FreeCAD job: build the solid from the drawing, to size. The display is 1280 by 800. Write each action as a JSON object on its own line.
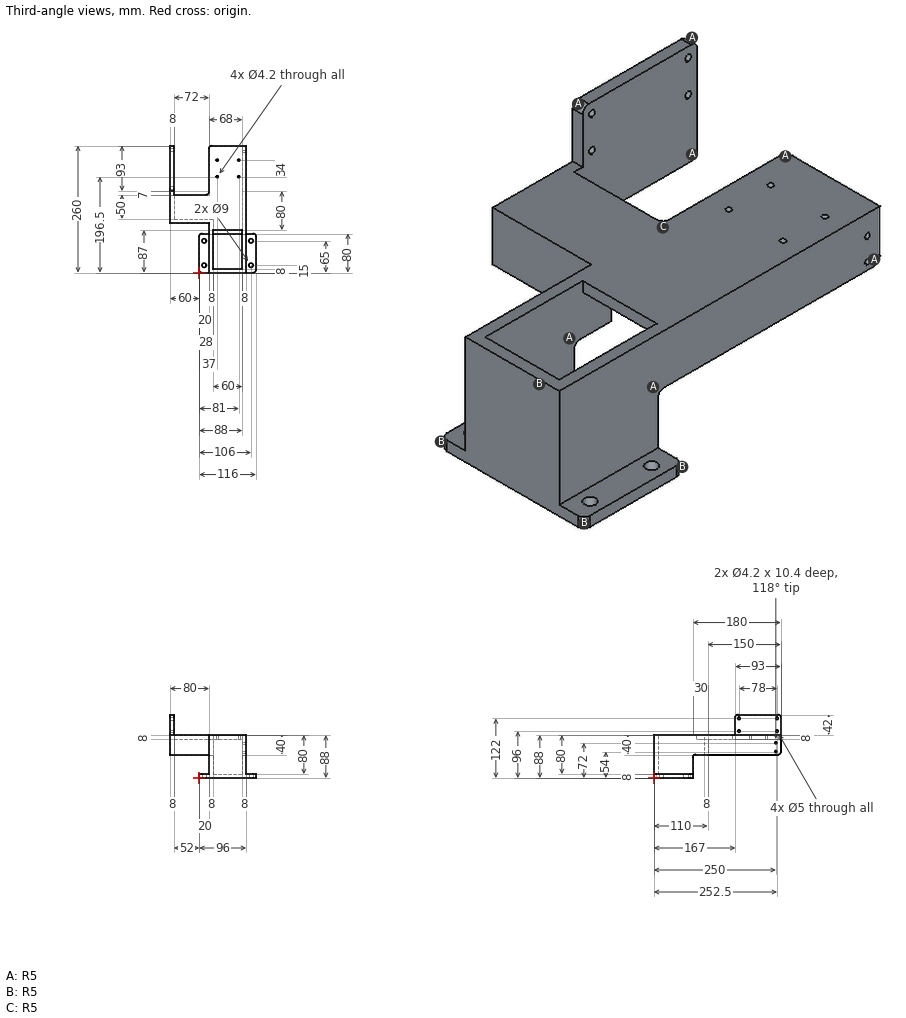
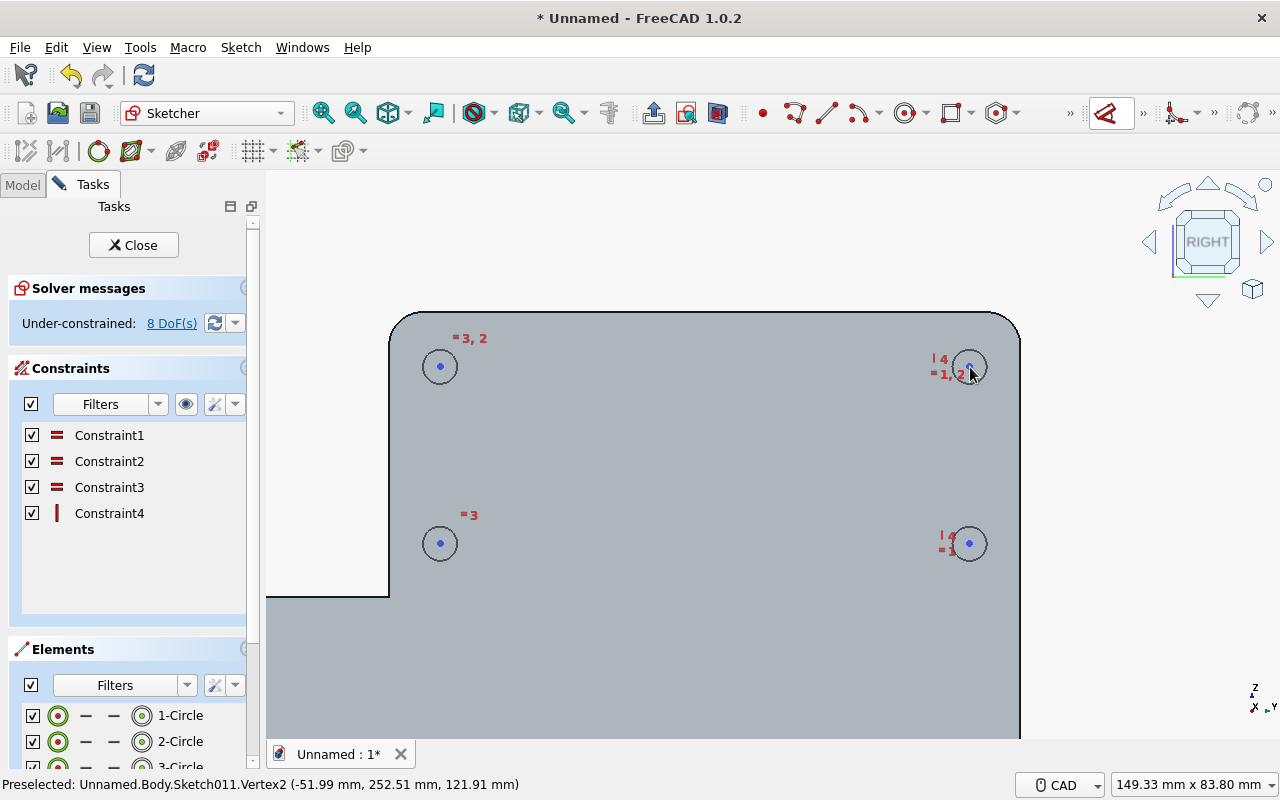
{"action": "left_click", "coordinate": [970, 367]}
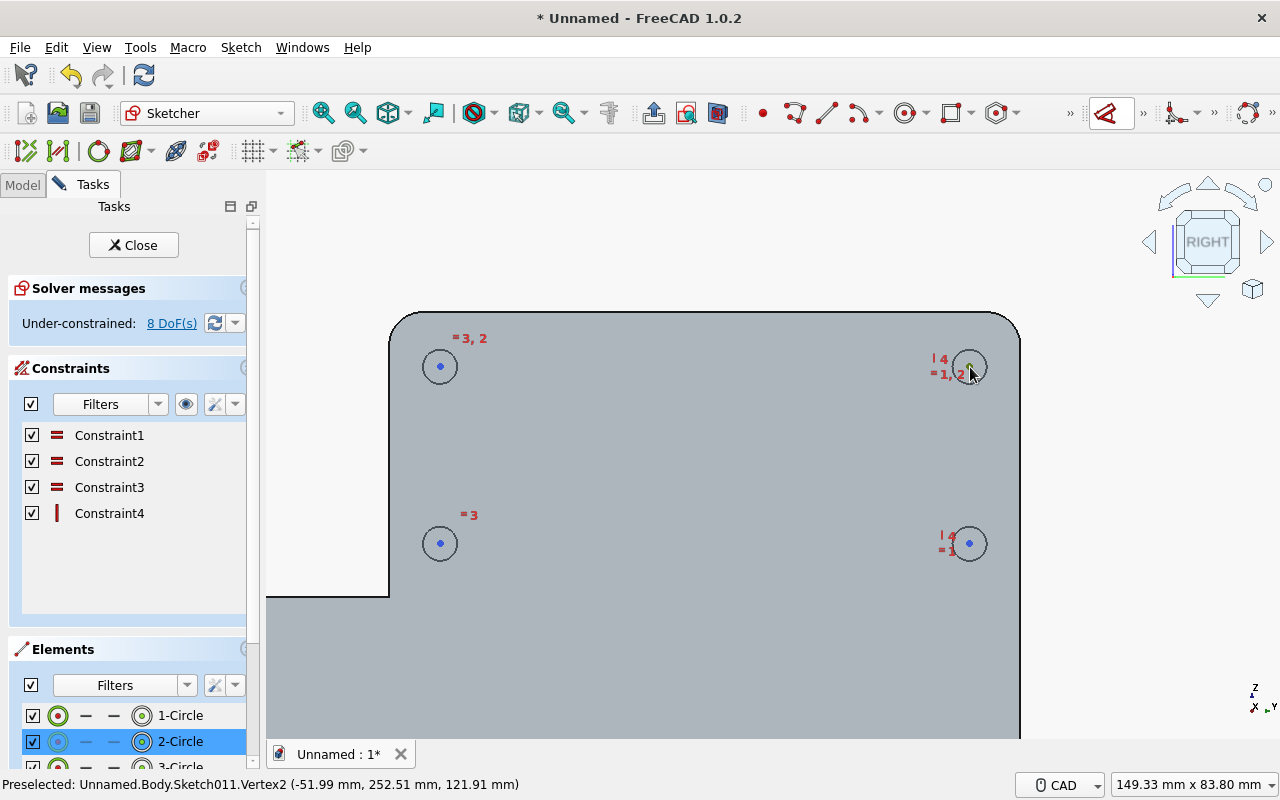
{"action": "left_click", "coordinate": [440, 367]}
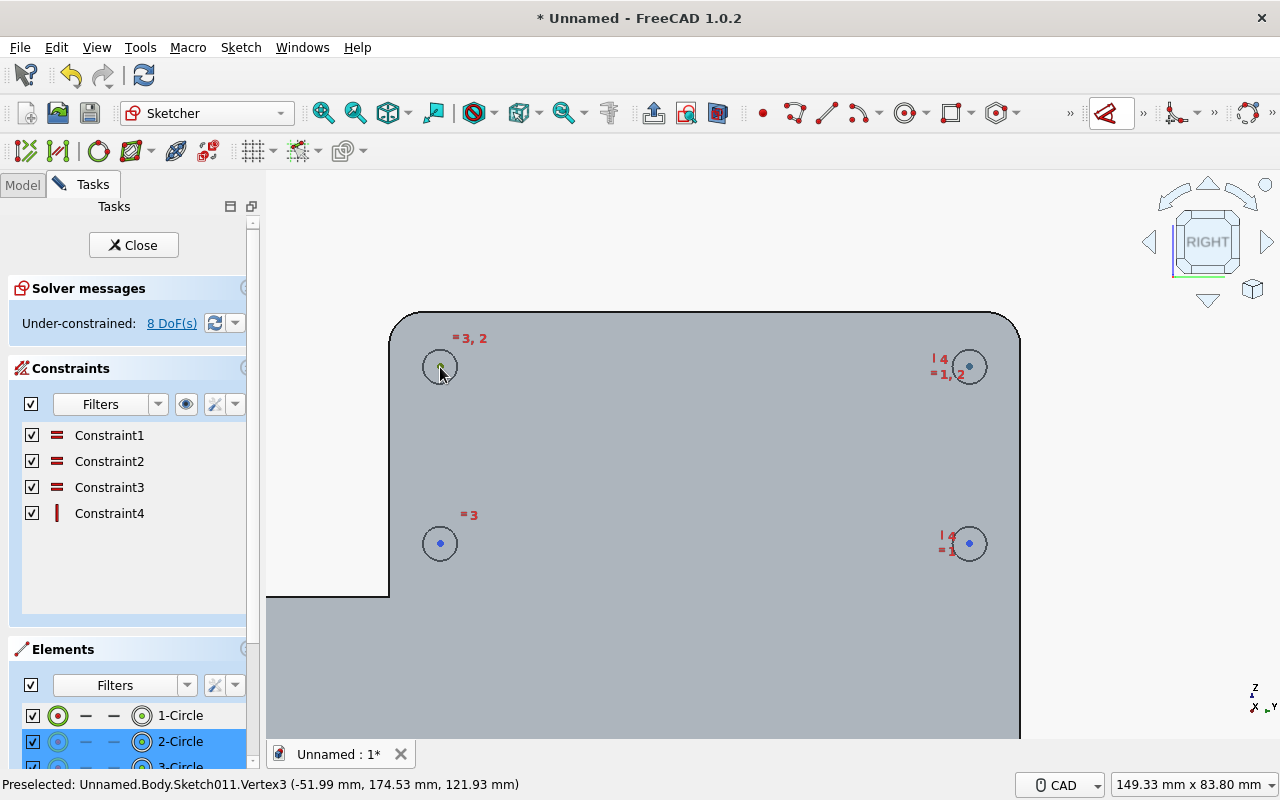
{"action": "key", "text": "h"}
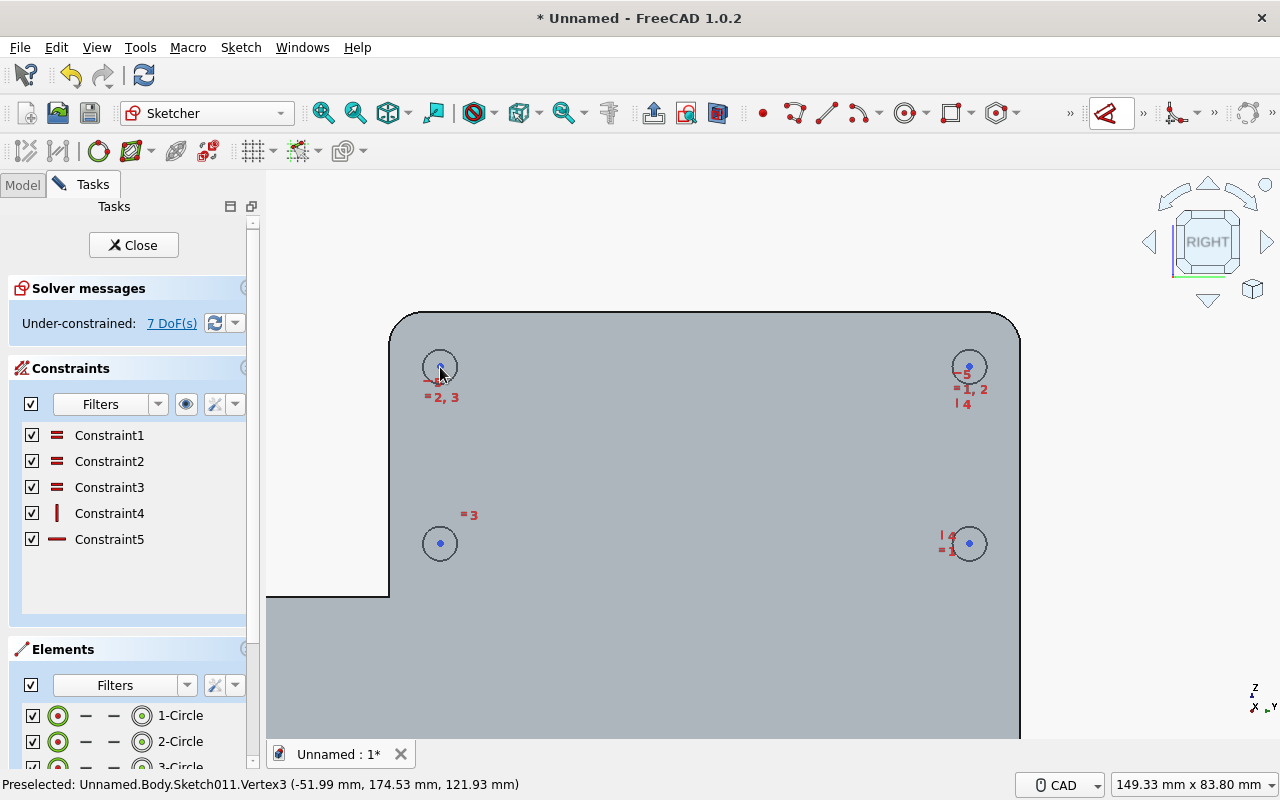
{"action": "left_click", "coordinate": [440, 367]}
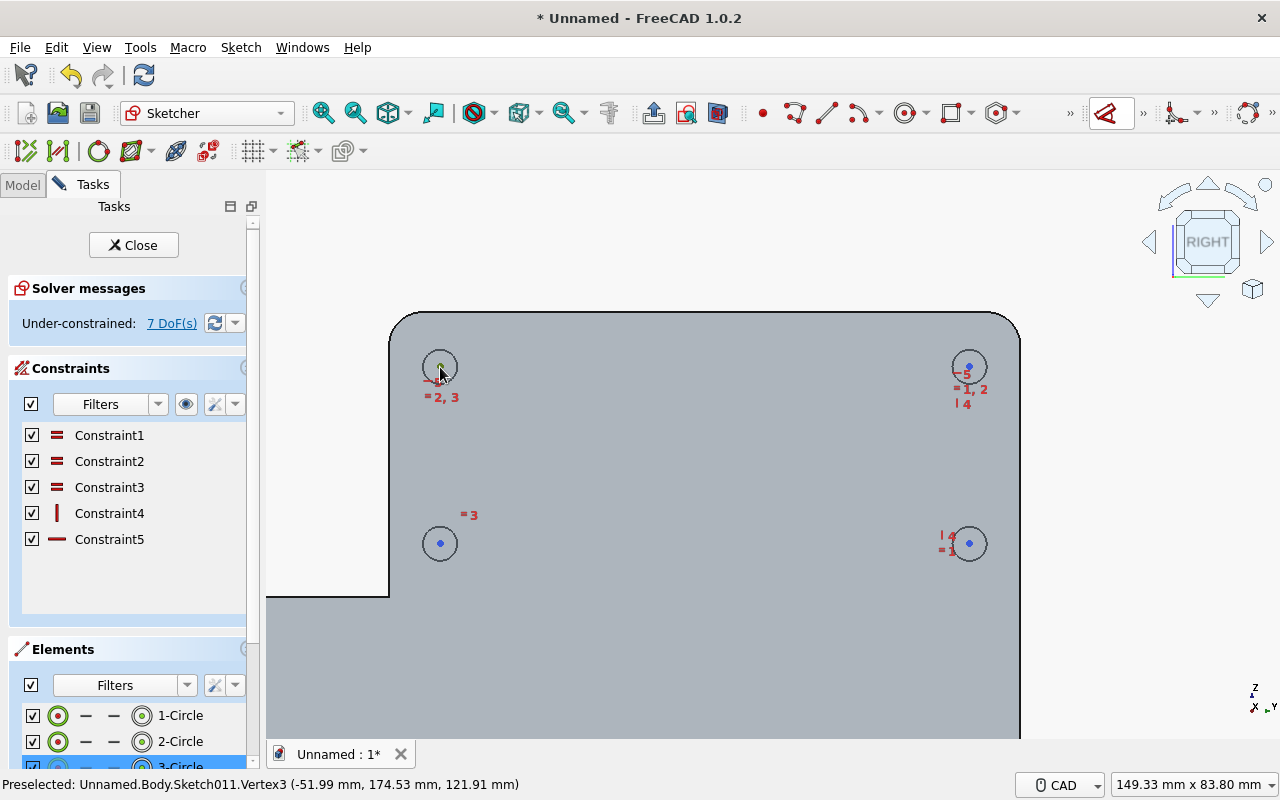
{"action": "left_click", "coordinate": [440, 544]}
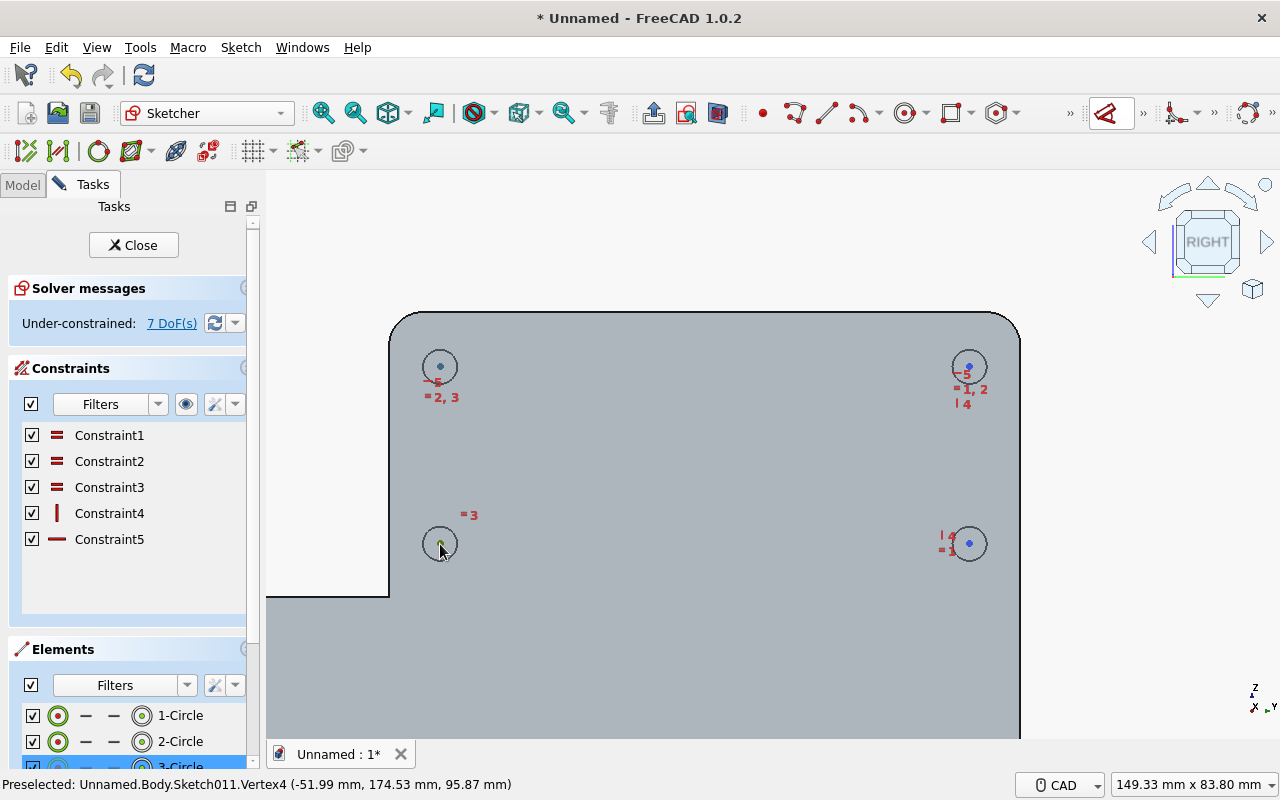
{"action": "key", "text": "v"}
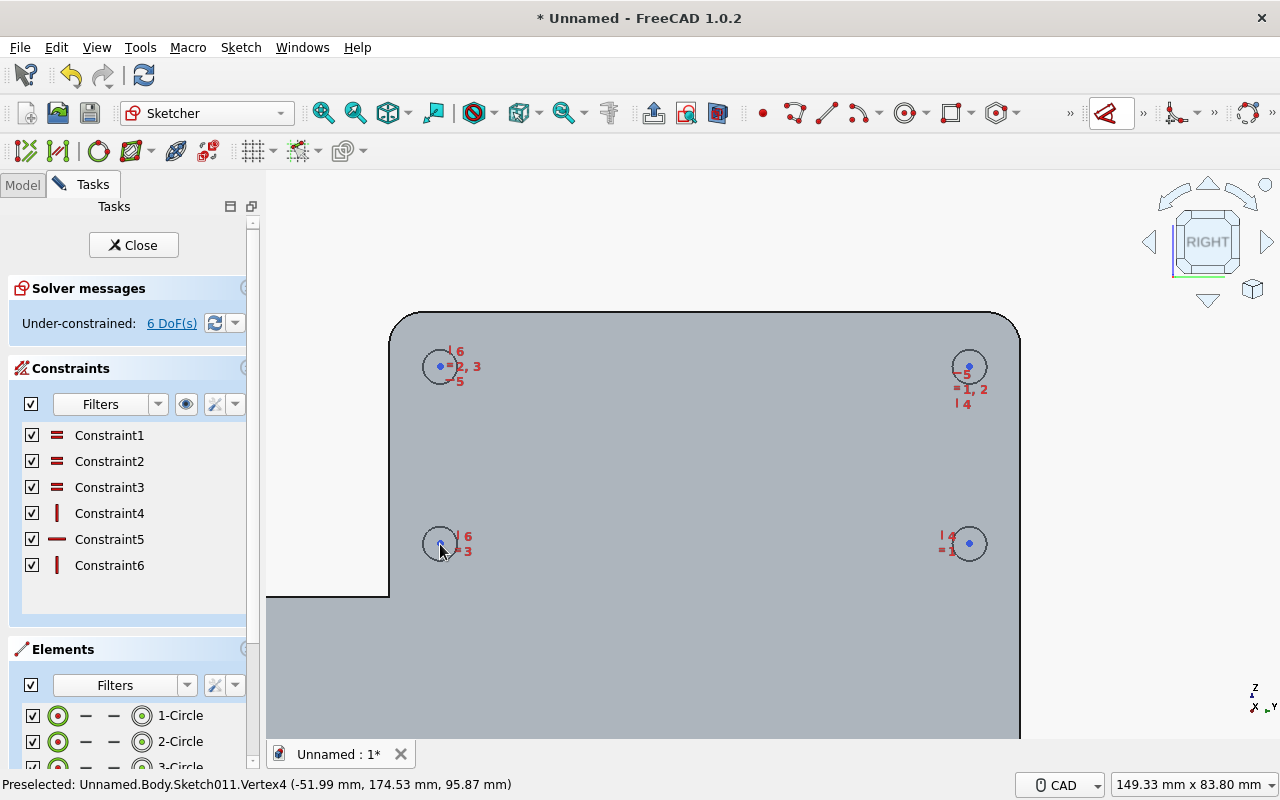
{"action": "left_click", "coordinate": [970, 544]}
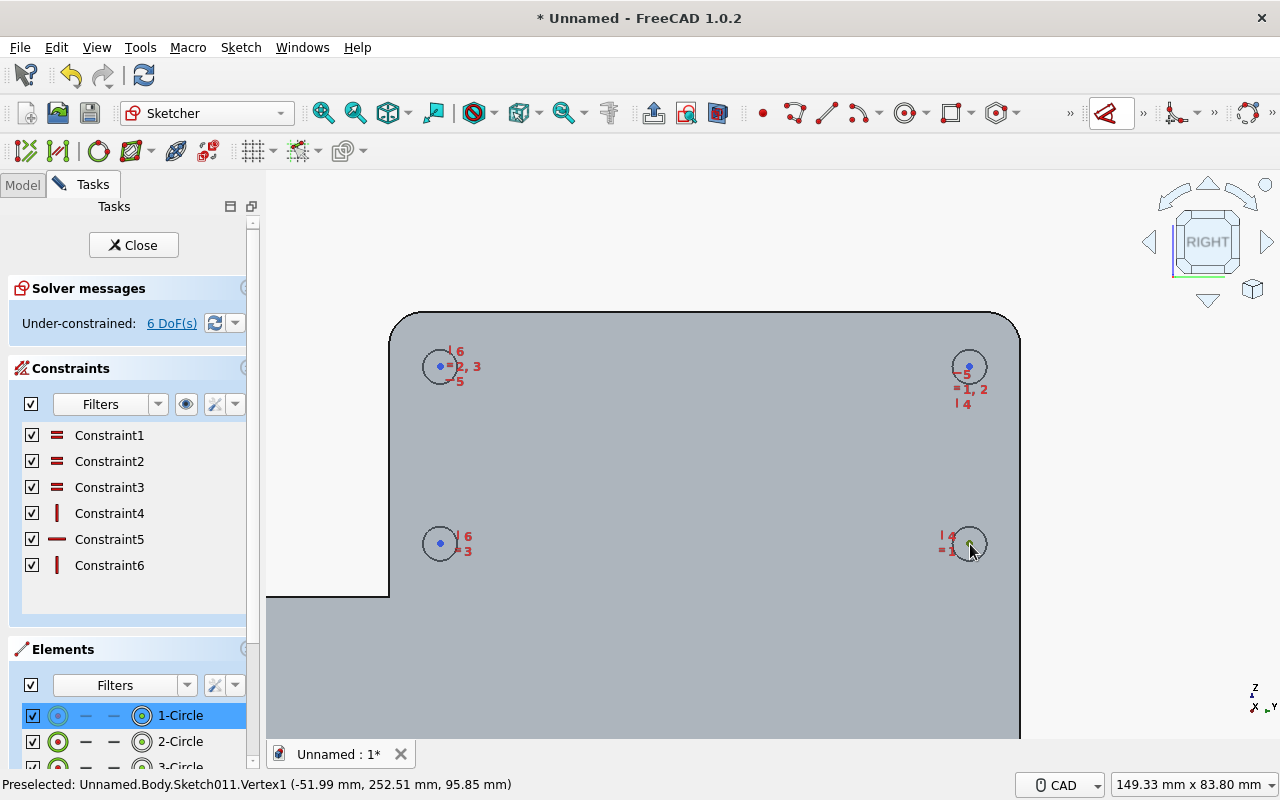
{"action": "left_click", "coordinate": [440, 544]}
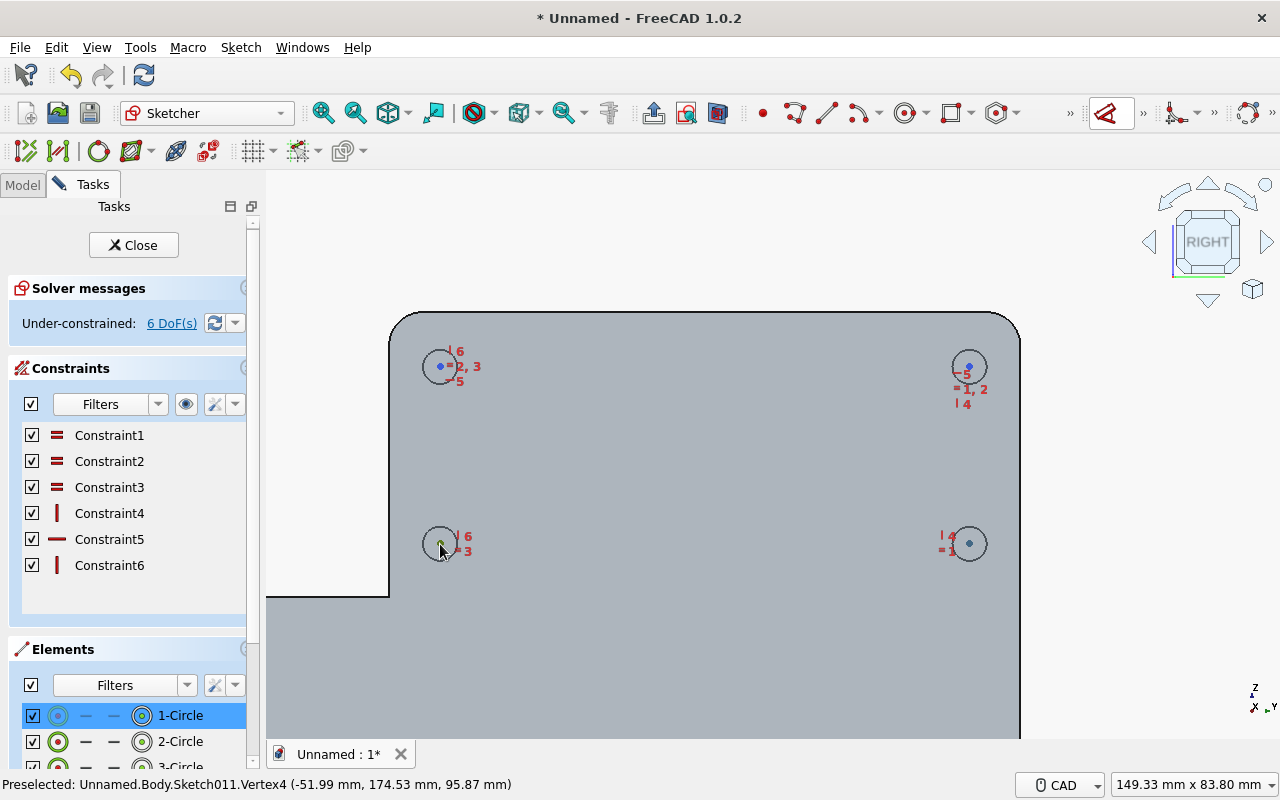
{"action": "key", "text": "h"}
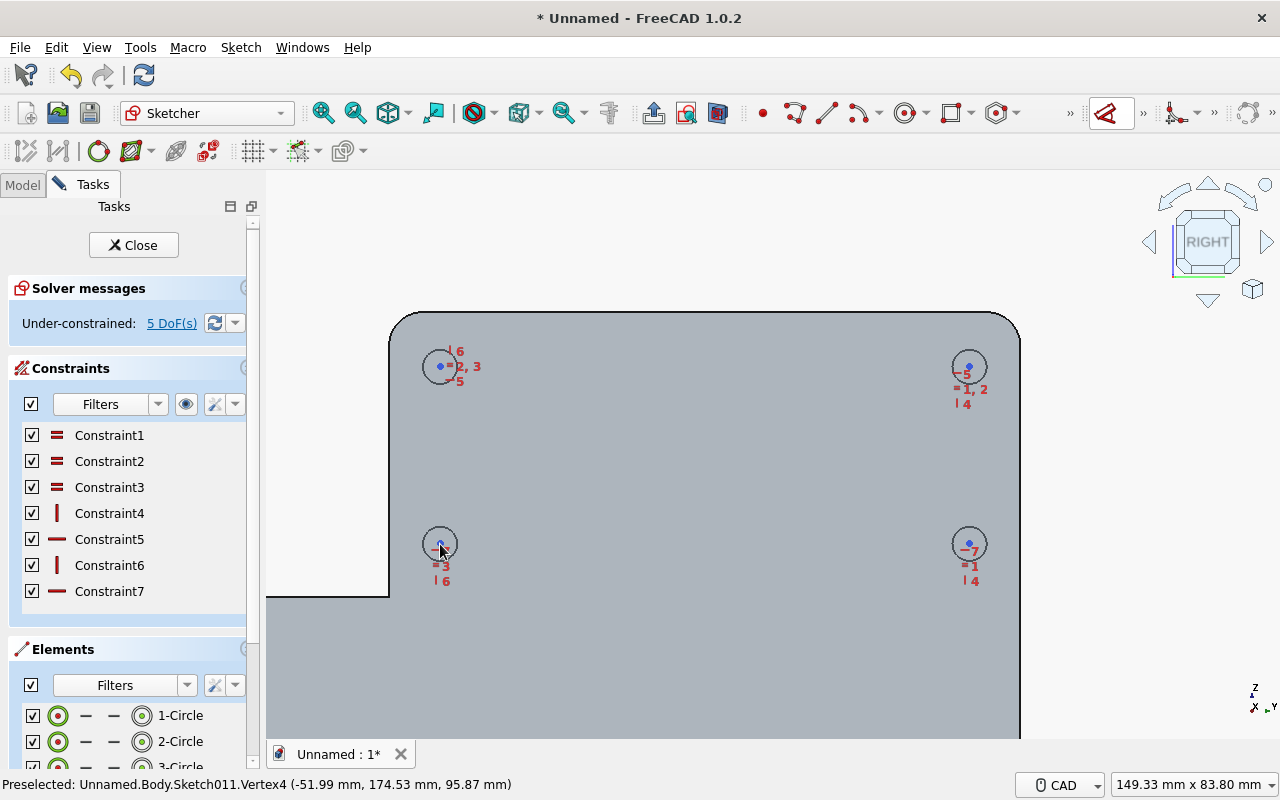
{"action": "left_click", "coordinate": [982, 532]}